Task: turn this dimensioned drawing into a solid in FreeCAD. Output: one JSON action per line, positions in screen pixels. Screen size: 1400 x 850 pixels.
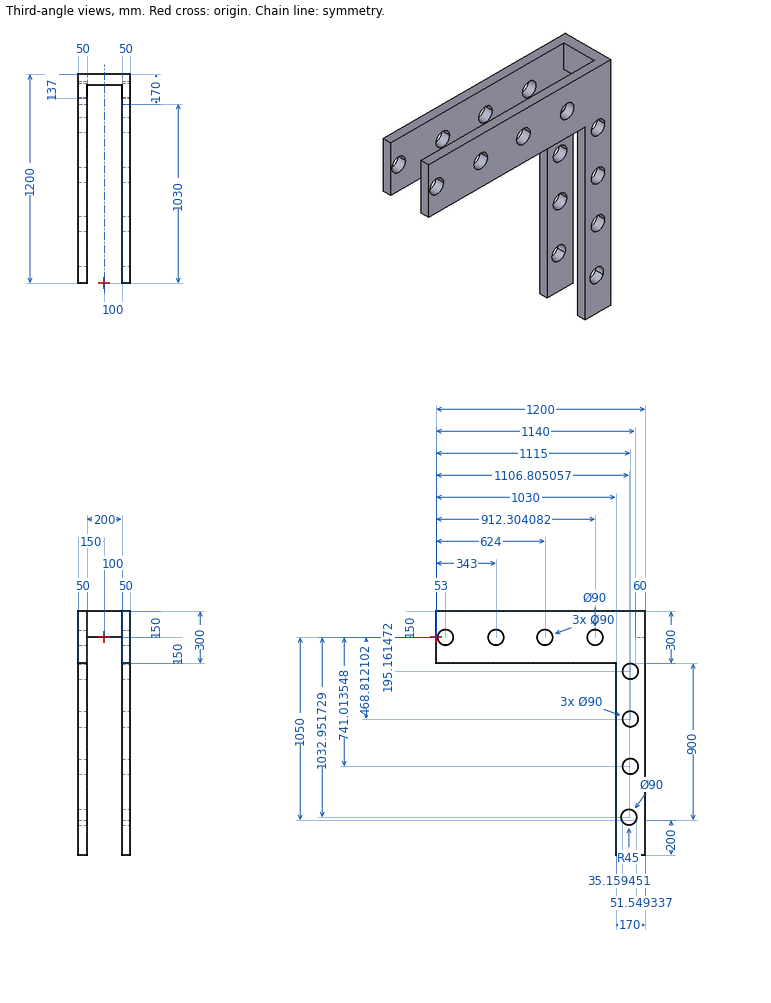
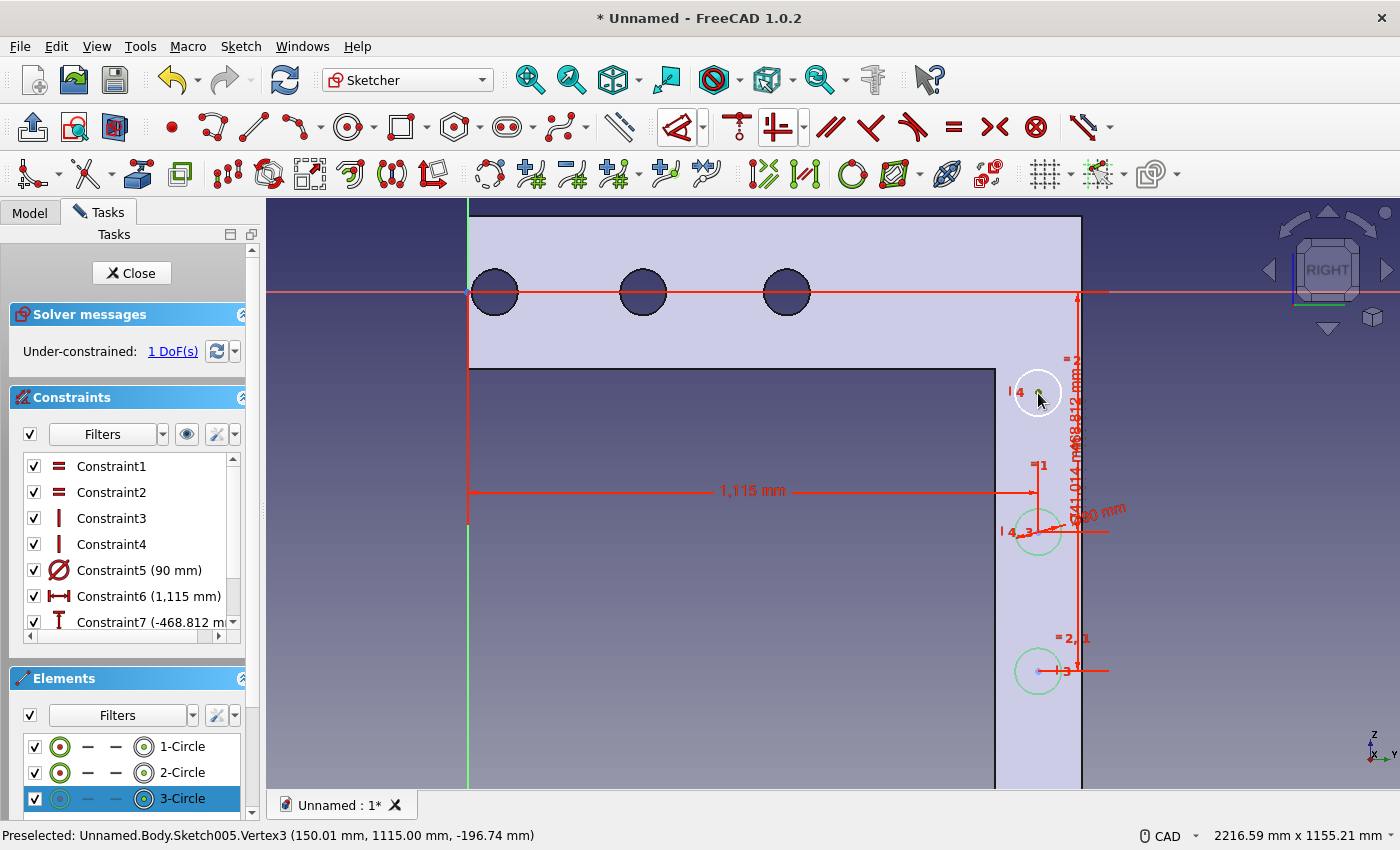
{"action": "key", "text": "i"}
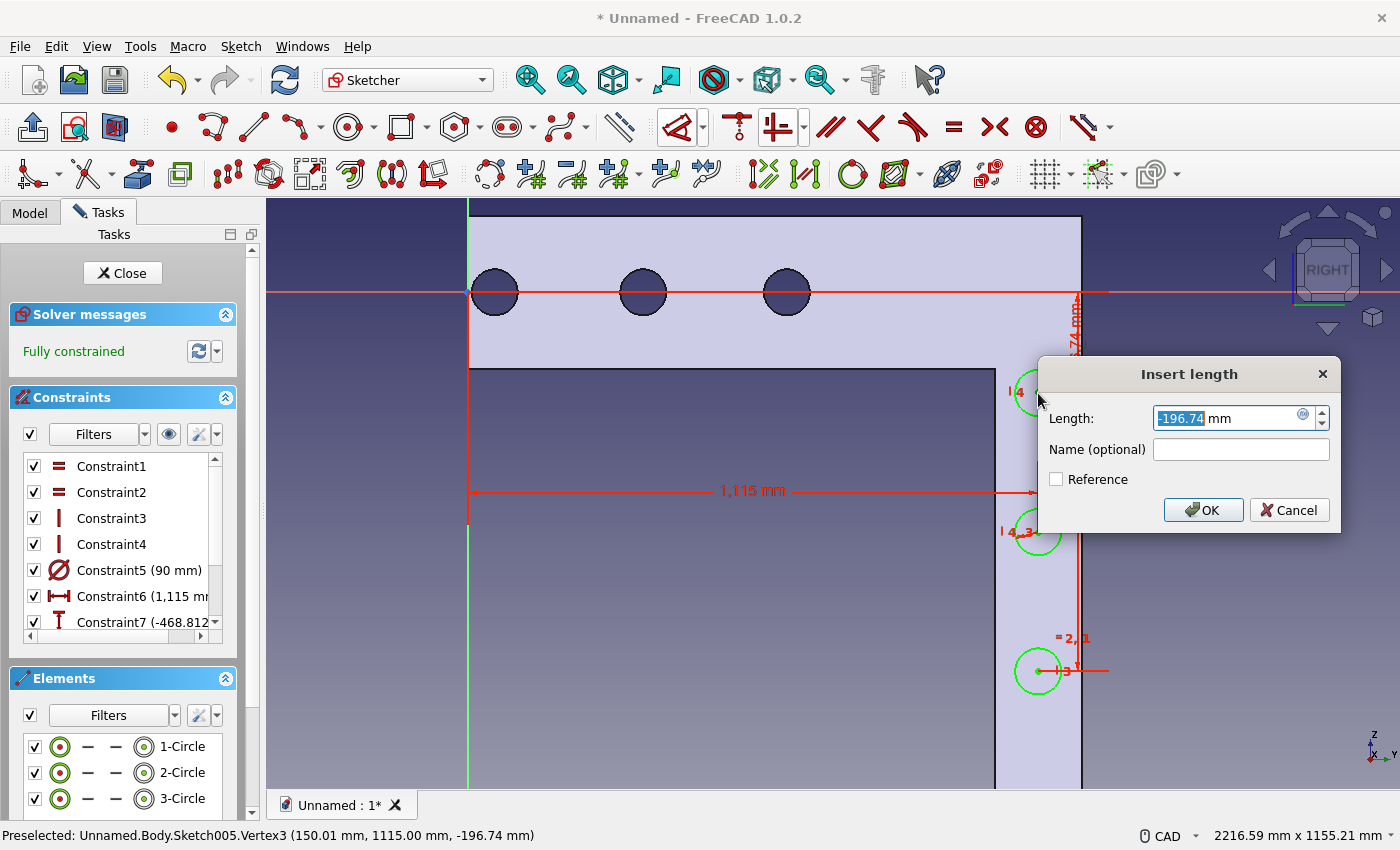
{"action": "type", "text": "-195.161472"}
{"action": "key", "text": "Return"}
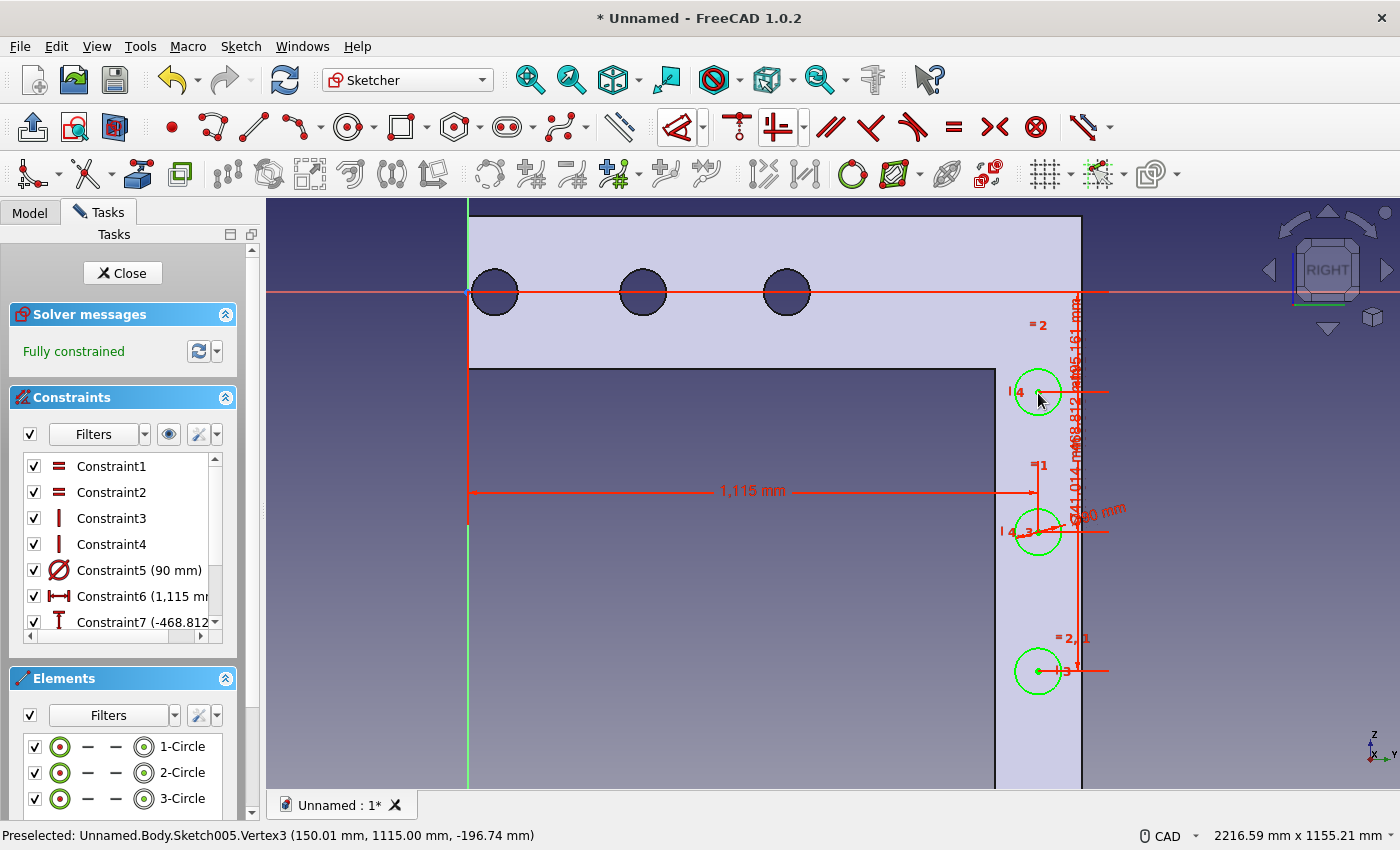
{"action": "left_click", "coordinate": [123, 273]}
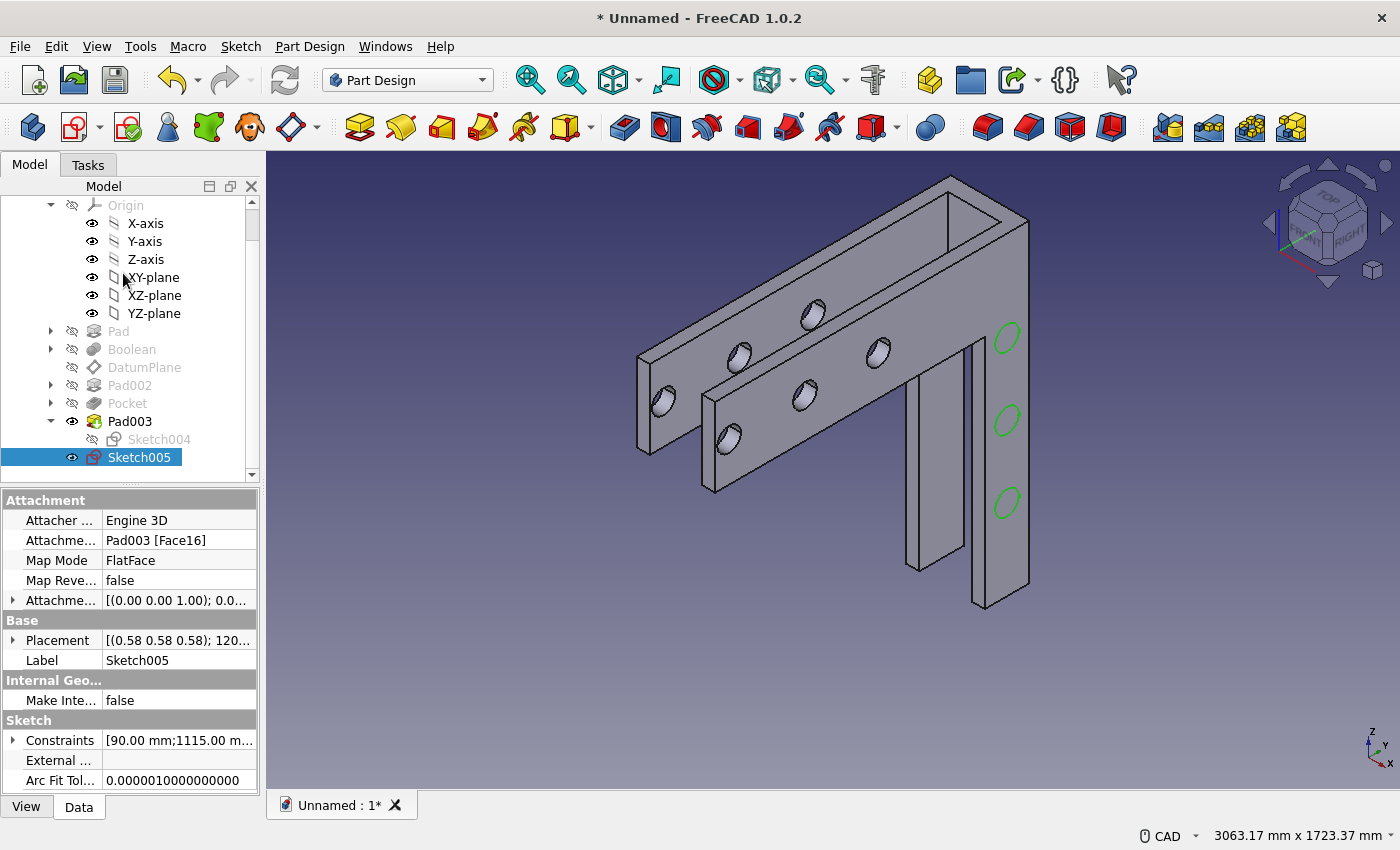
{"action": "left_click", "coordinate": [625, 128]}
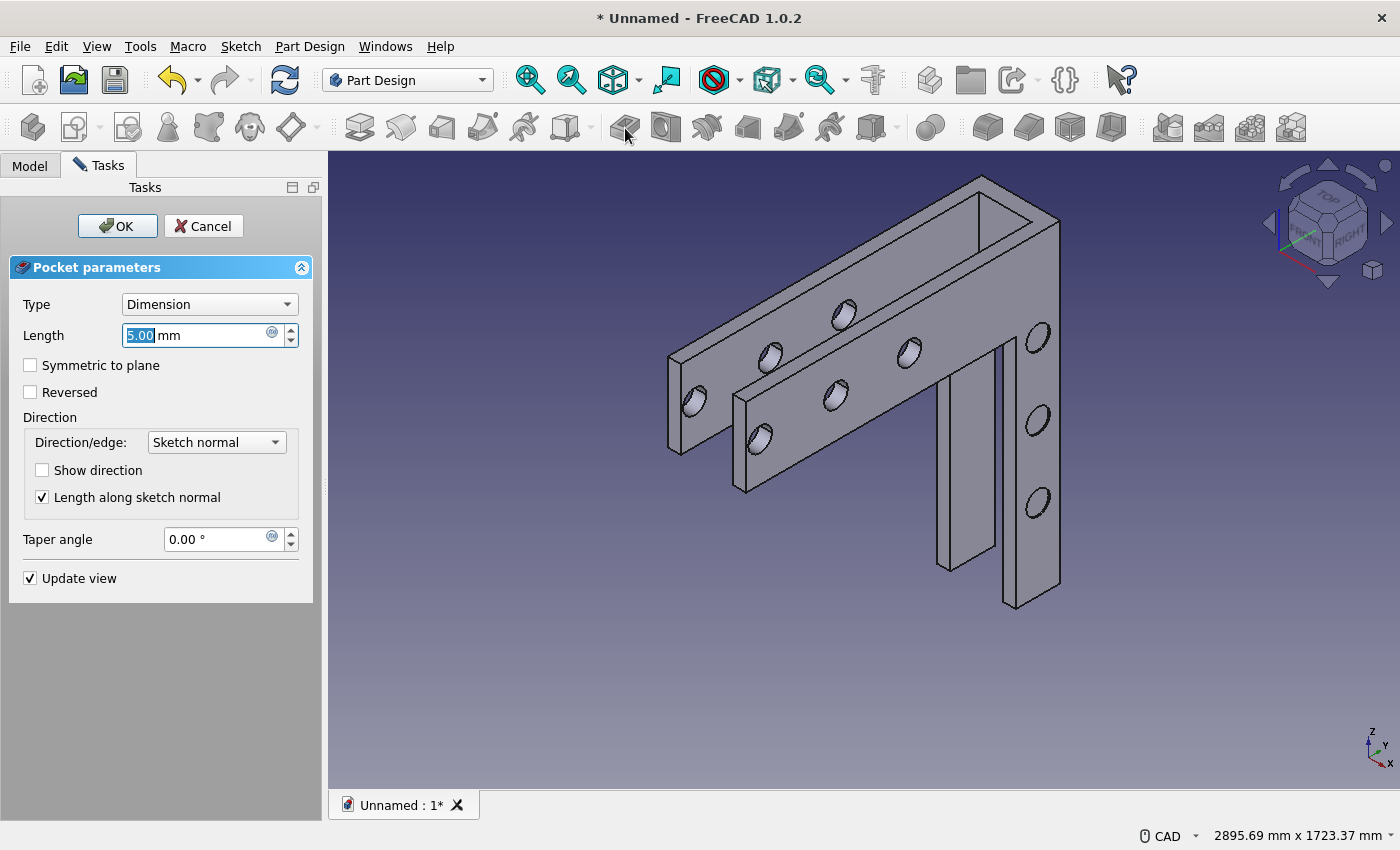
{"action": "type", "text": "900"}
{"action": "key", "text": "Tab"}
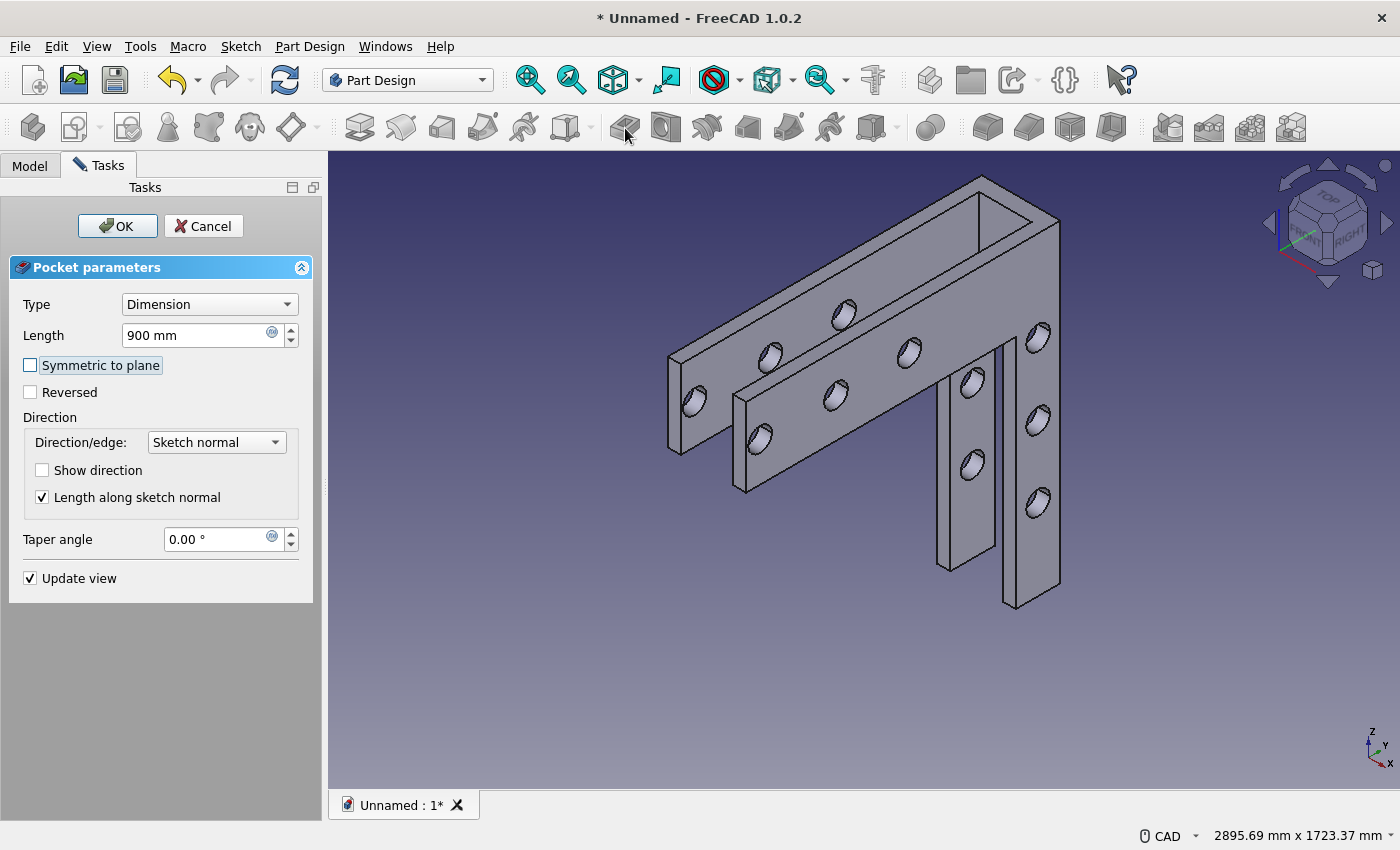
{"action": "left_click", "coordinate": [118, 226]}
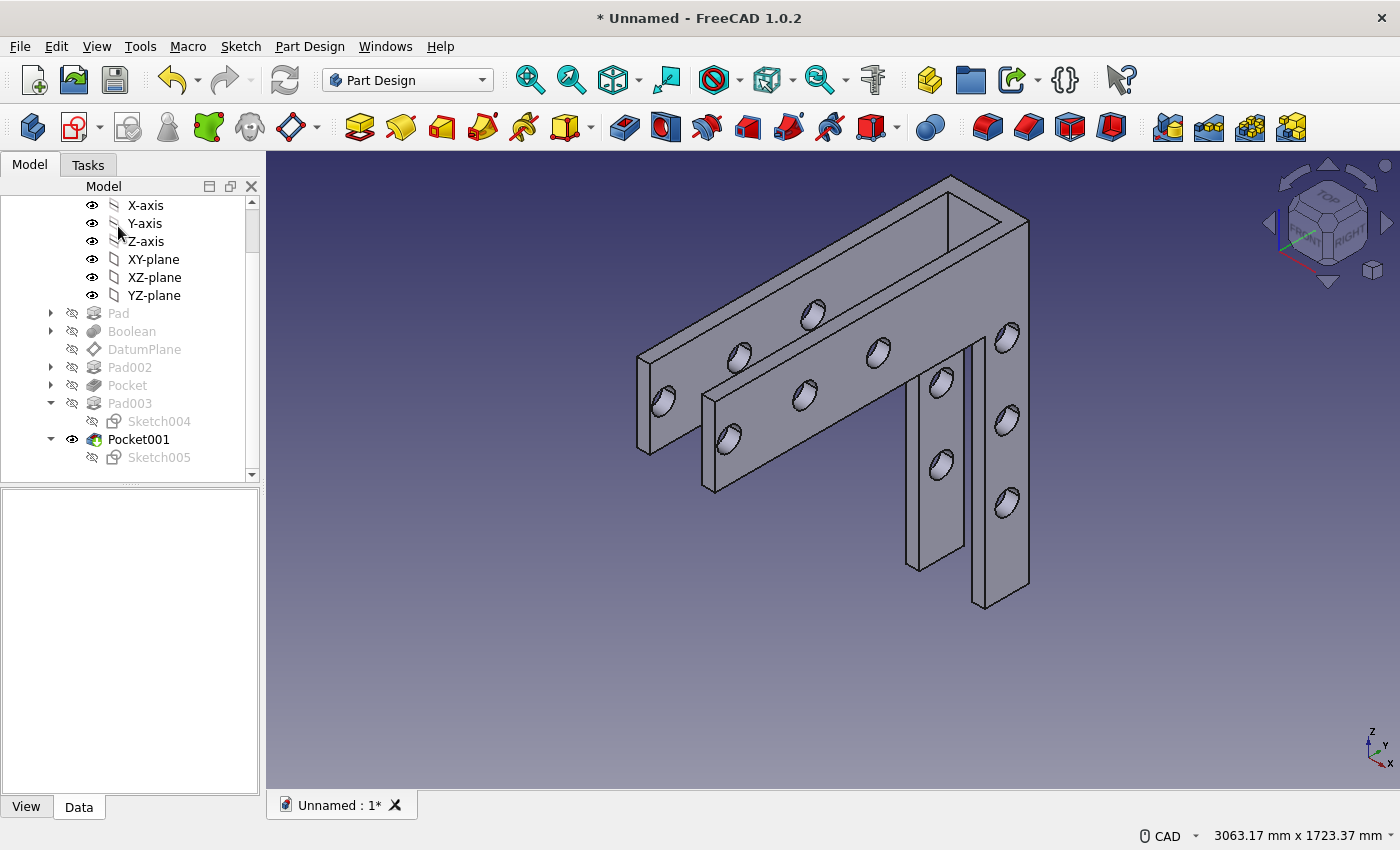
{"action": "key", "text": "4"}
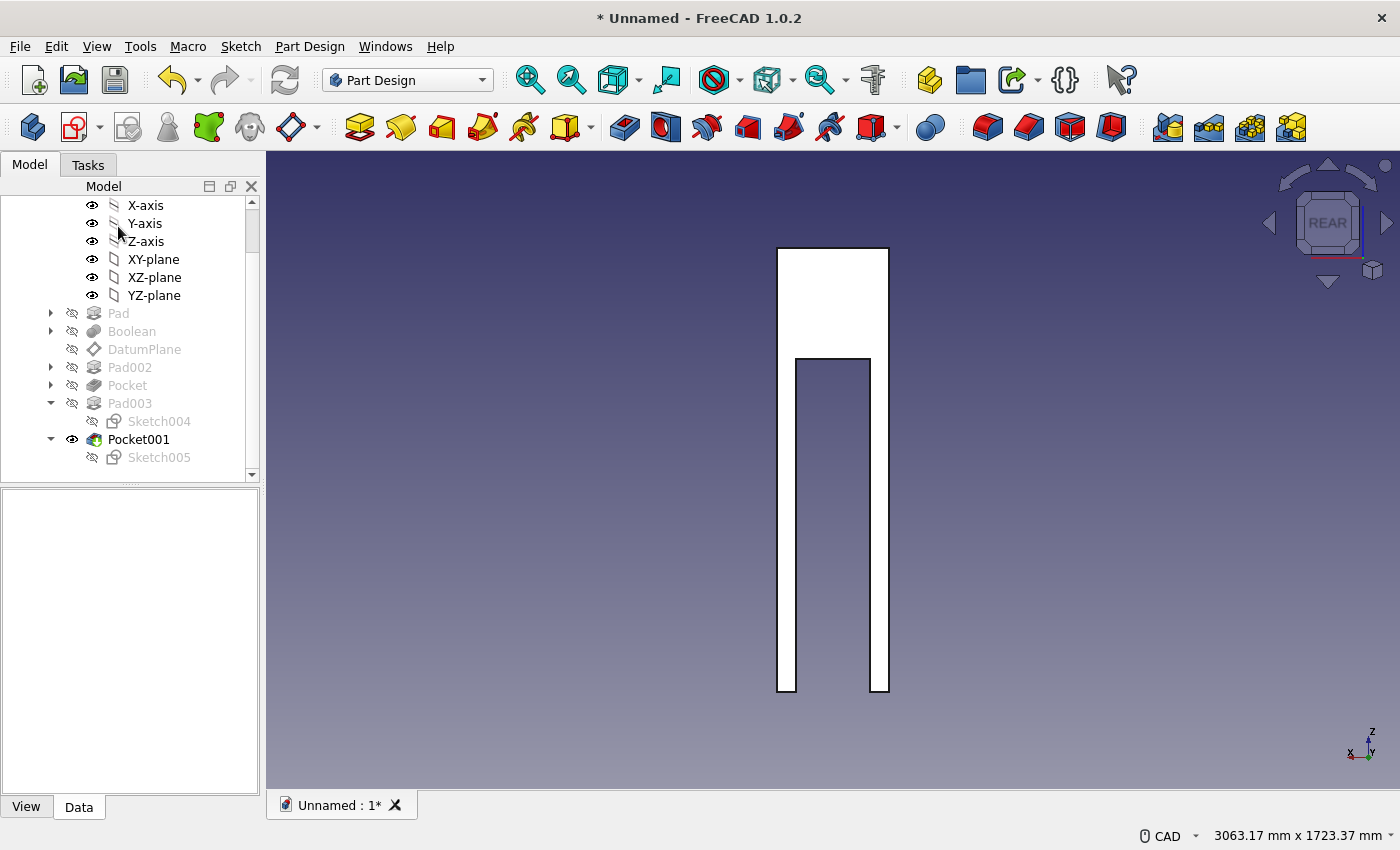
{"action": "left_click", "coordinate": [817, 279]}